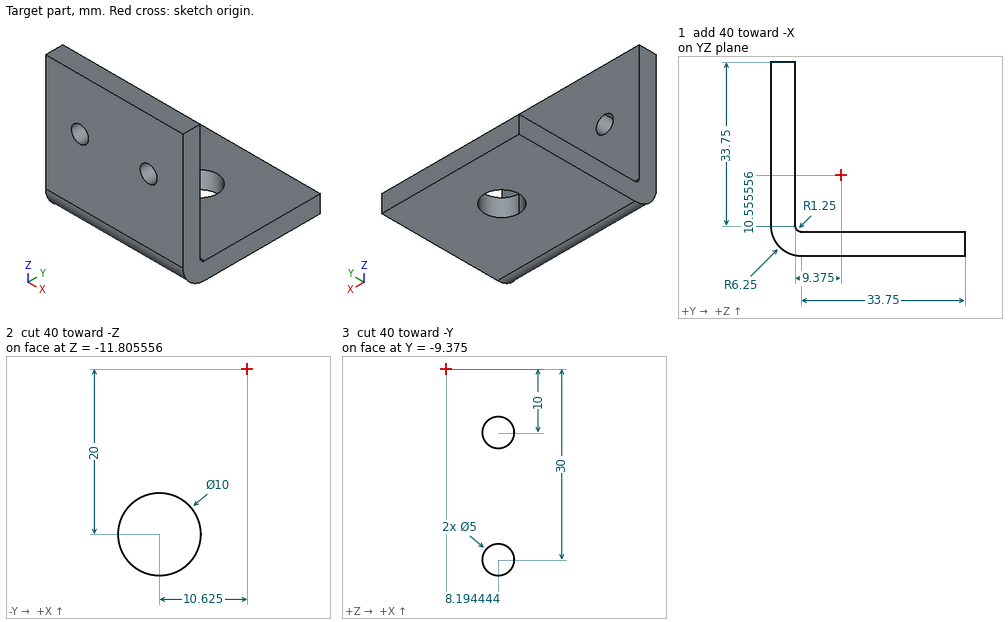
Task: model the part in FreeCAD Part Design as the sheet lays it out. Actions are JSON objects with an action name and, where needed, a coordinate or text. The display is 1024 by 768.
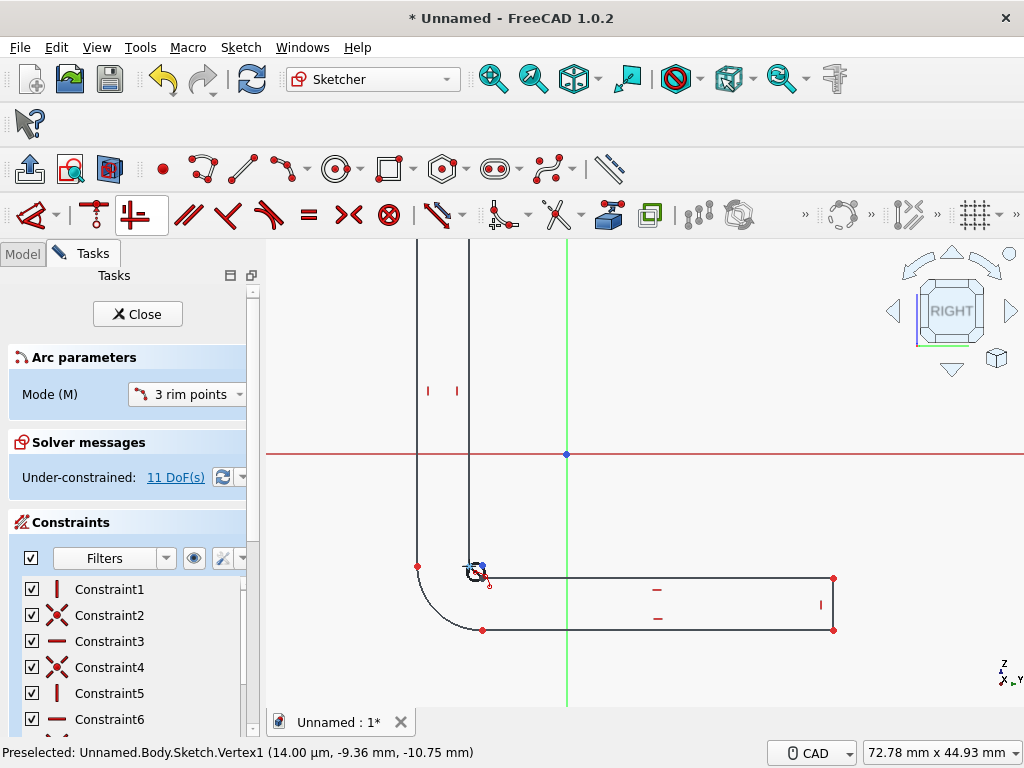
{"action": "scroll", "coordinate": [473, 573], "scroll_direction": "up", "scroll_amount": 8}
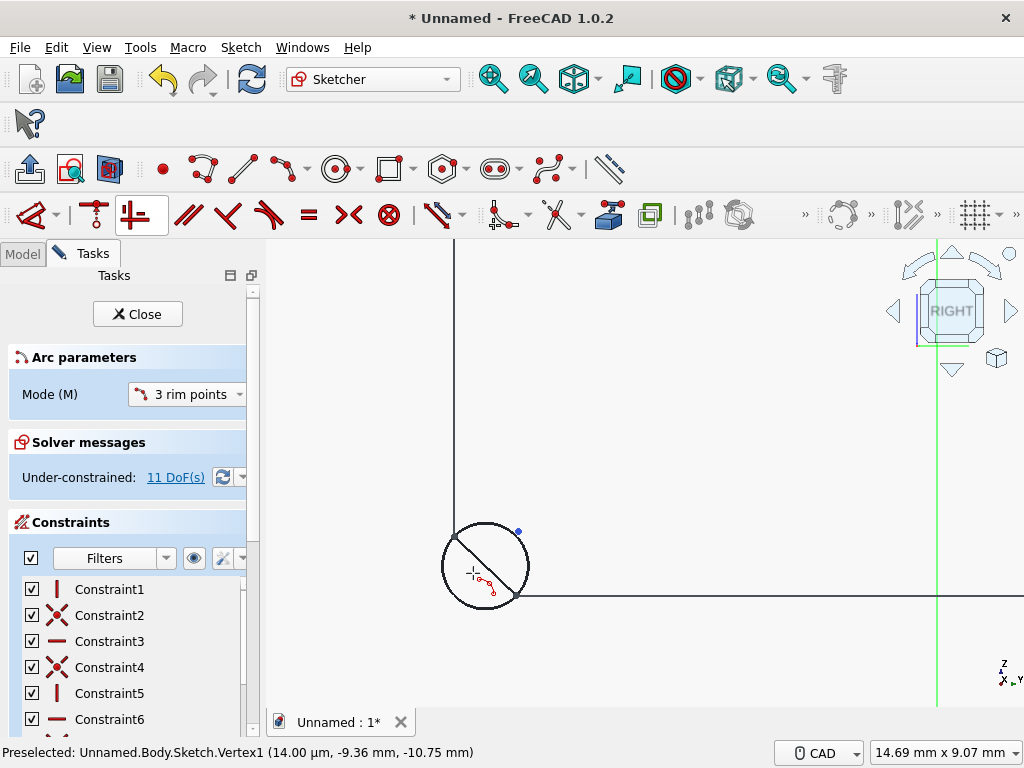
{"action": "left_click", "coordinate": [472, 572]}
{"action": "key", "text": "Escape"}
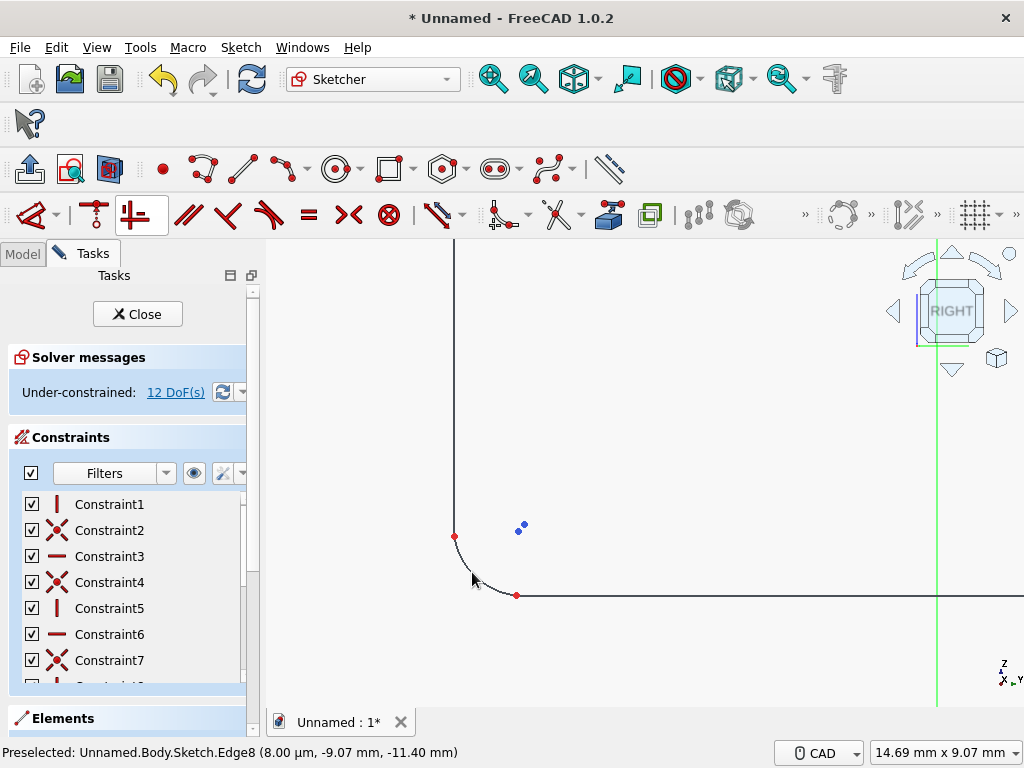
{"action": "scroll", "coordinate": [475, 576], "scroll_direction": "down", "scroll_amount": 10}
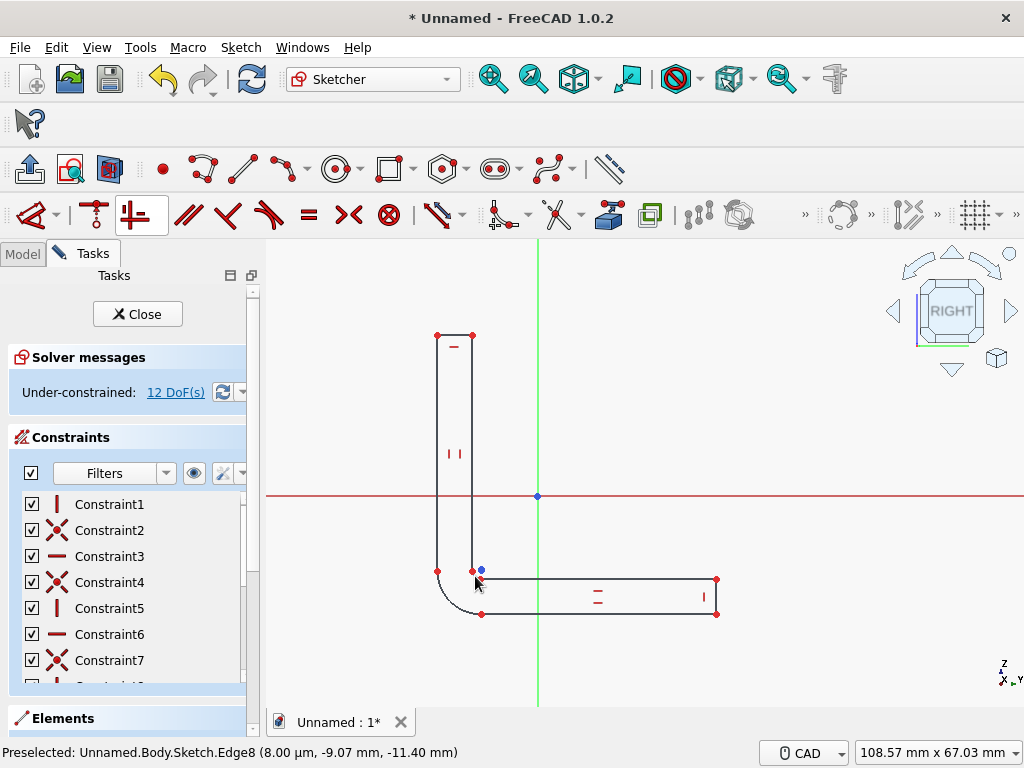
{"action": "scroll", "coordinate": [472, 500], "scroll_direction": "up", "scroll_amount": 6}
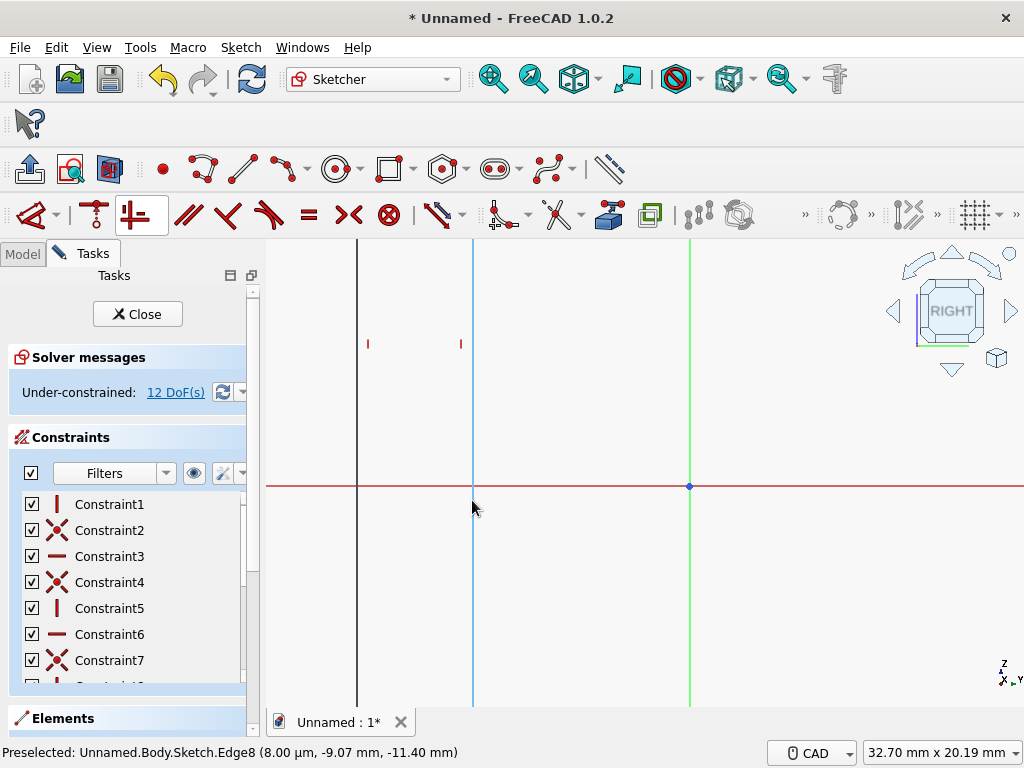
{"action": "left_click", "coordinate": [473, 500]}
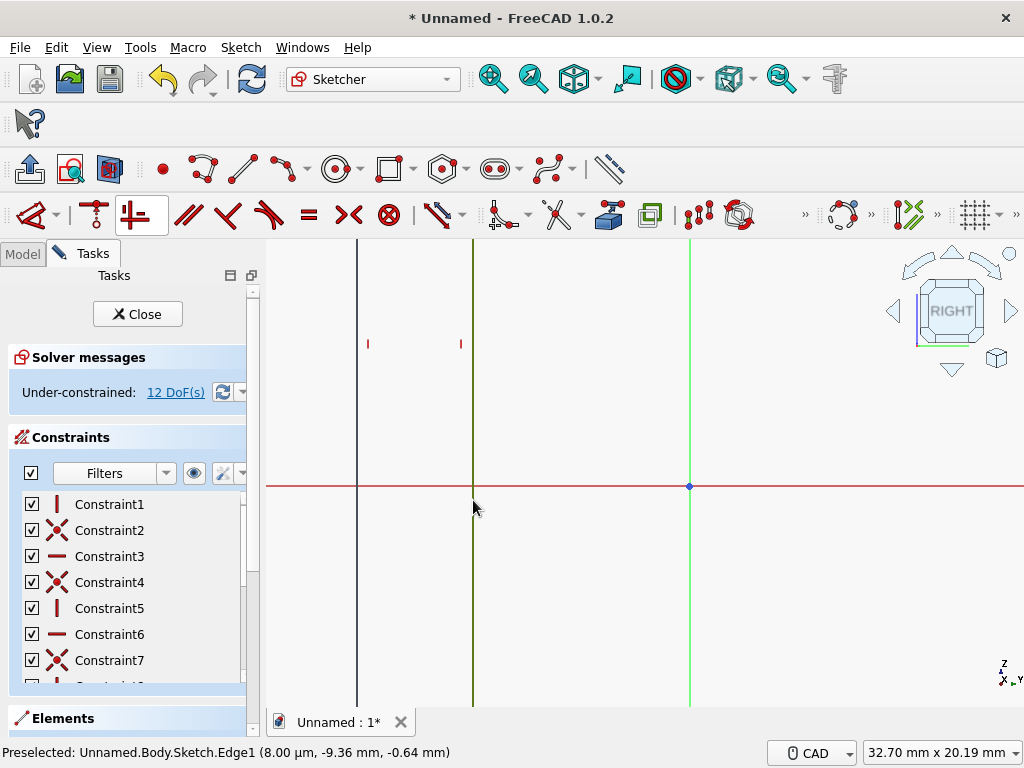
{"action": "scroll", "coordinate": [471, 499], "scroll_direction": "down", "scroll_amount": 6}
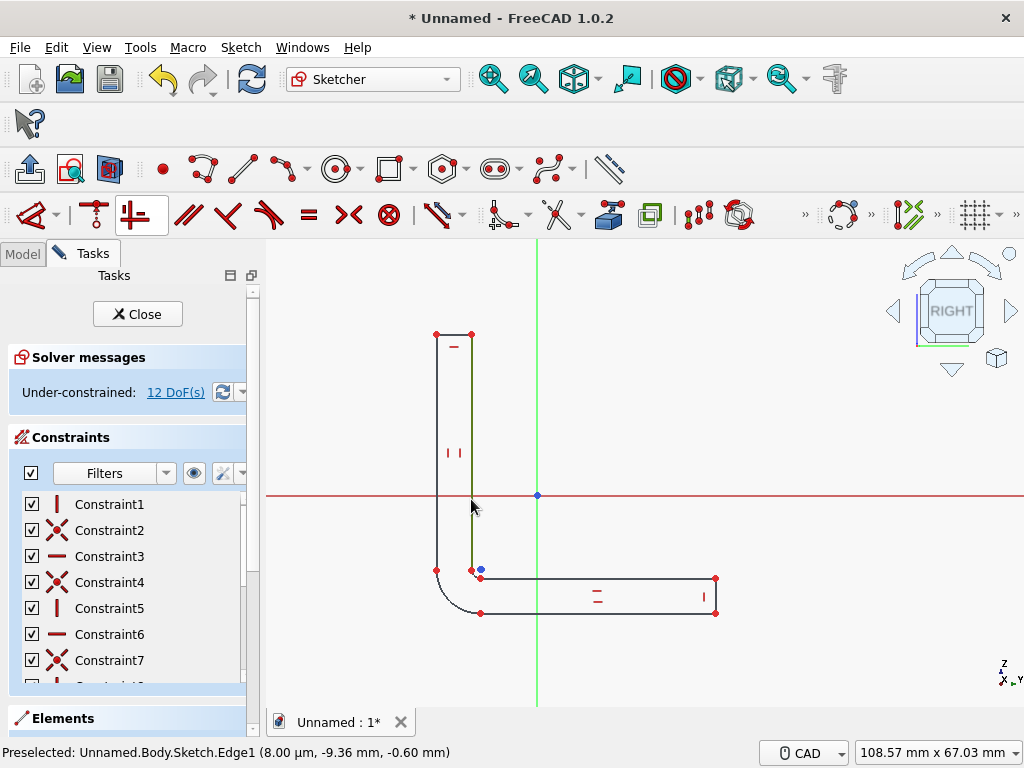
{"action": "scroll", "coordinate": [473, 574], "scroll_direction": "up", "scroll_amount": 7}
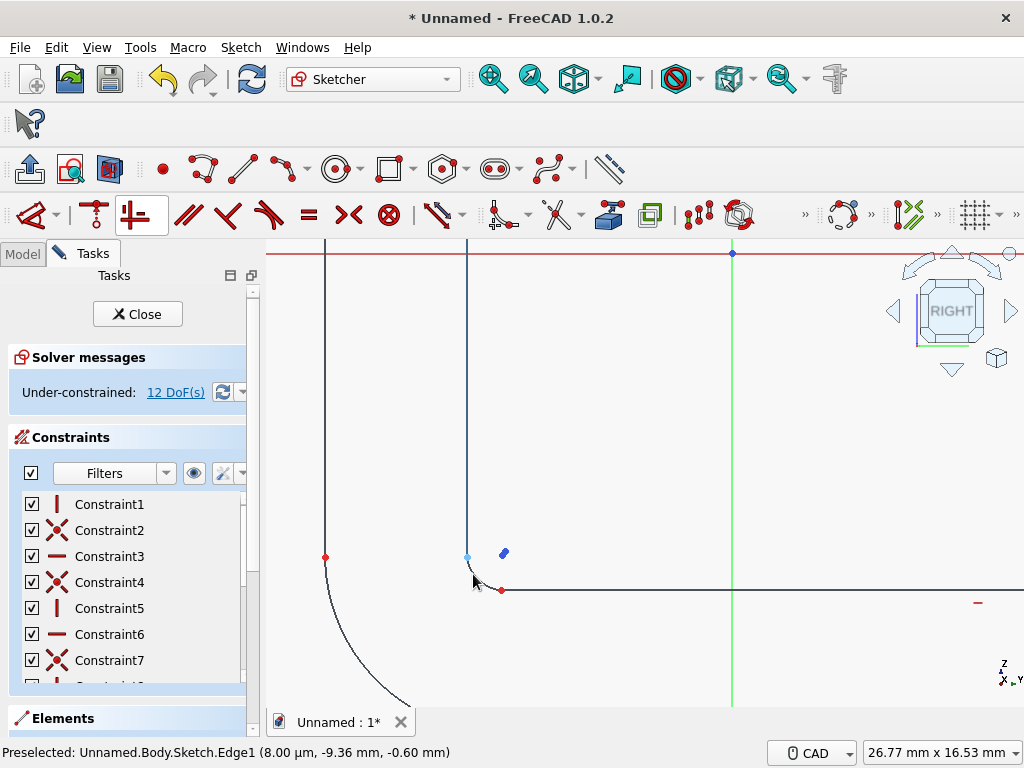
{"action": "left_click", "coordinate": [472, 572]}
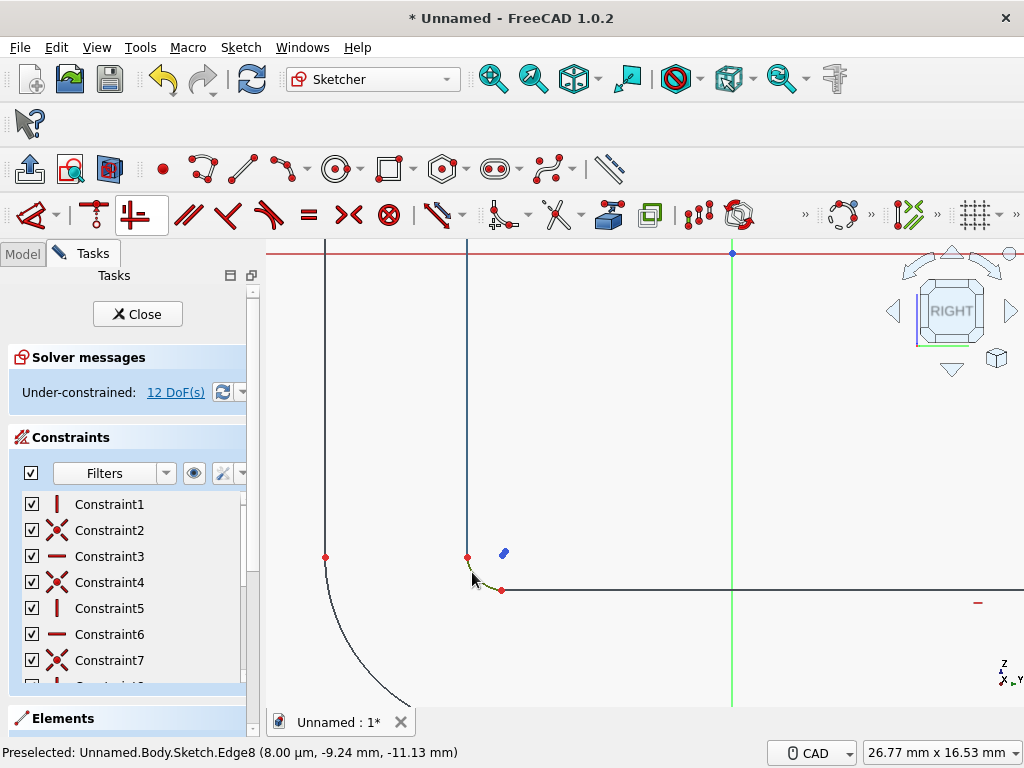
{"action": "key", "text": "t"}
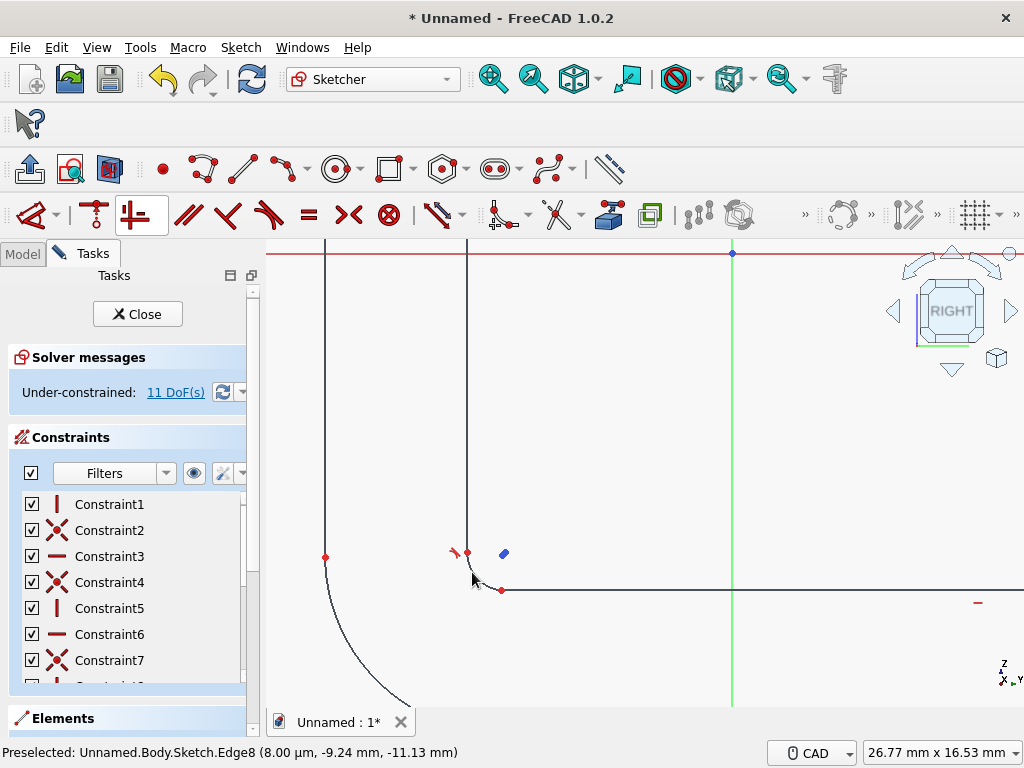
{"action": "left_click", "coordinate": [325, 271]}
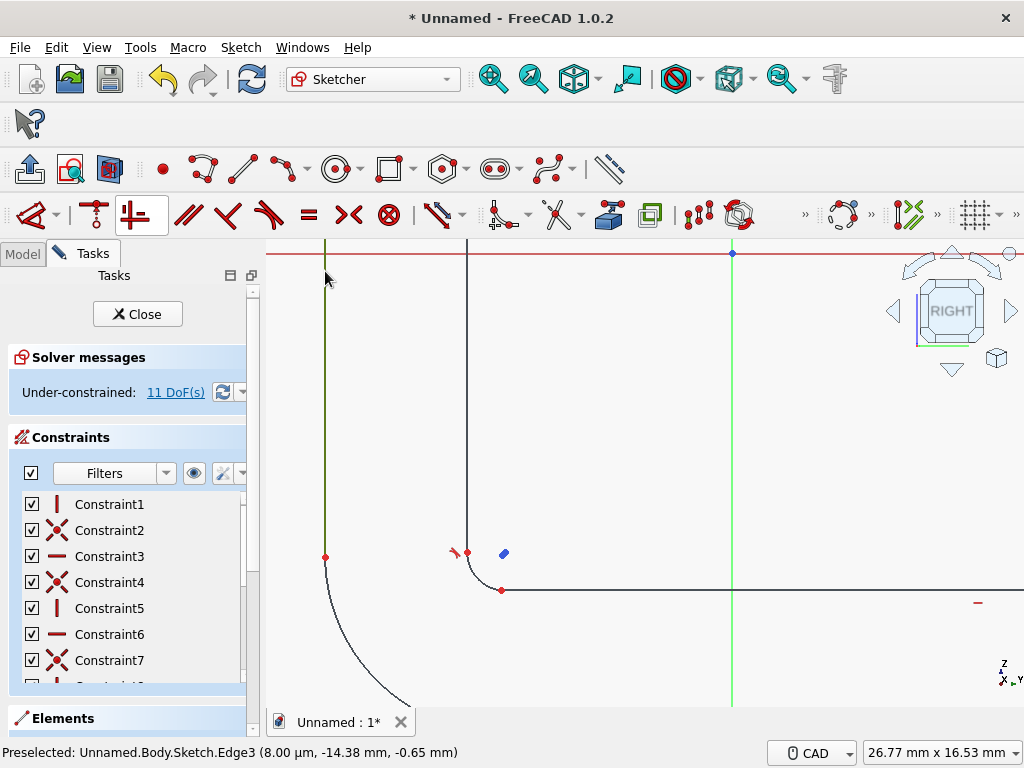
{"action": "scroll", "coordinate": [473, 574], "scroll_direction": "down", "scroll_amount": 7}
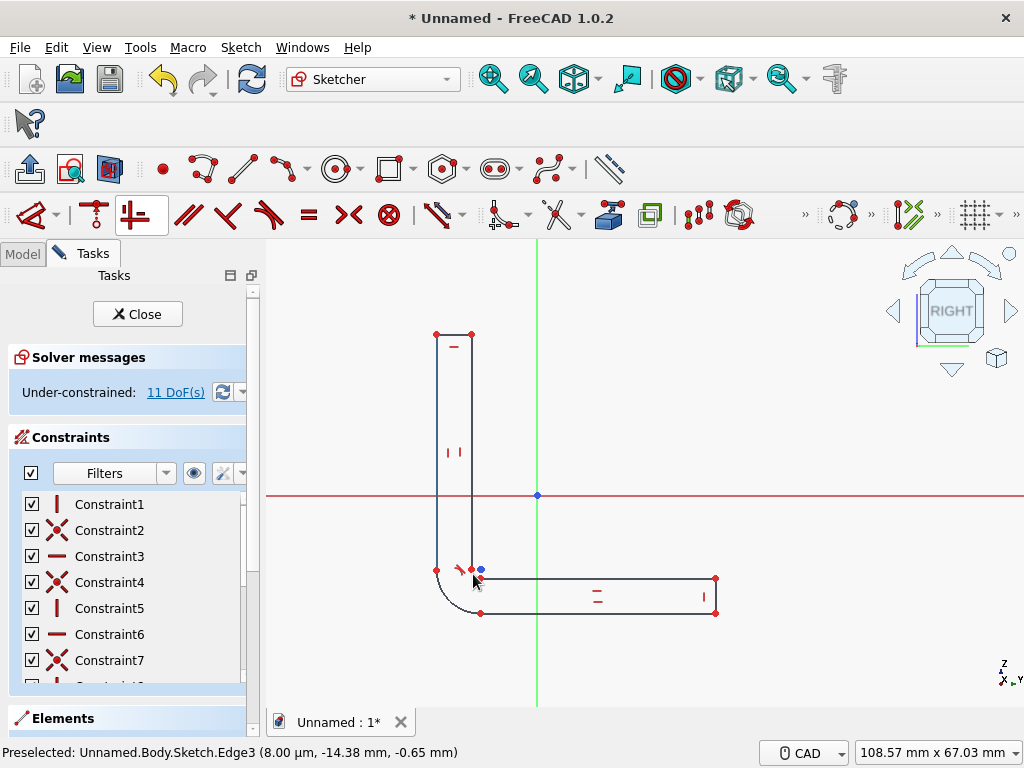
{"action": "left_click", "coordinate": [442, 590]}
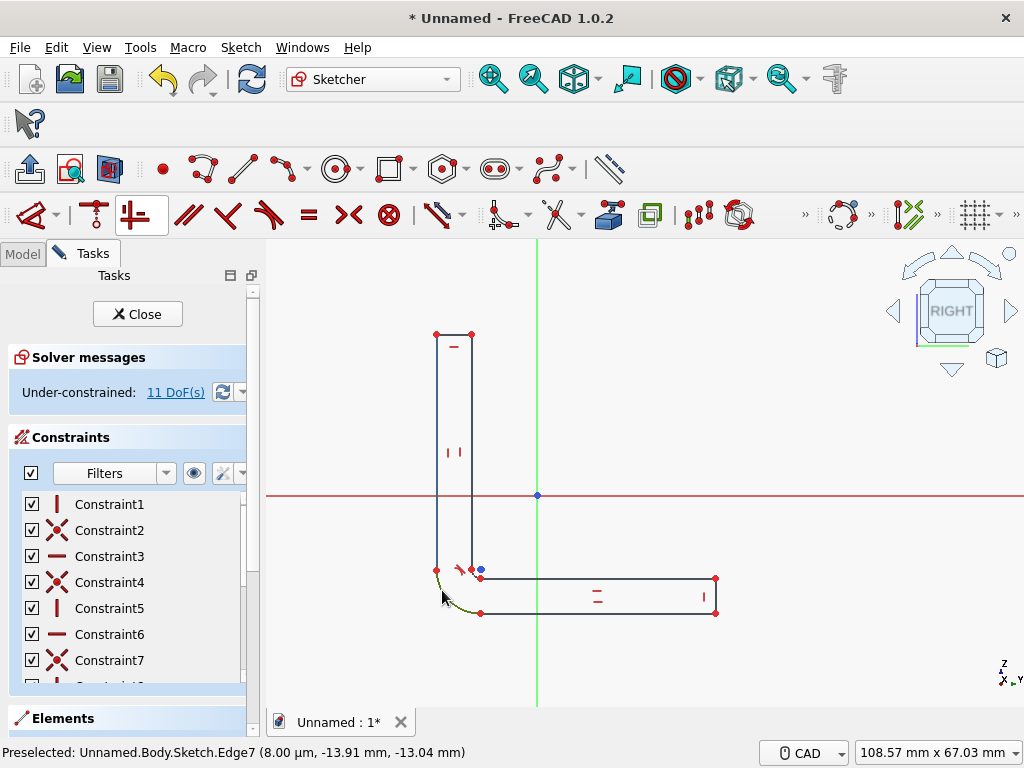
{"action": "key", "text": "t"}